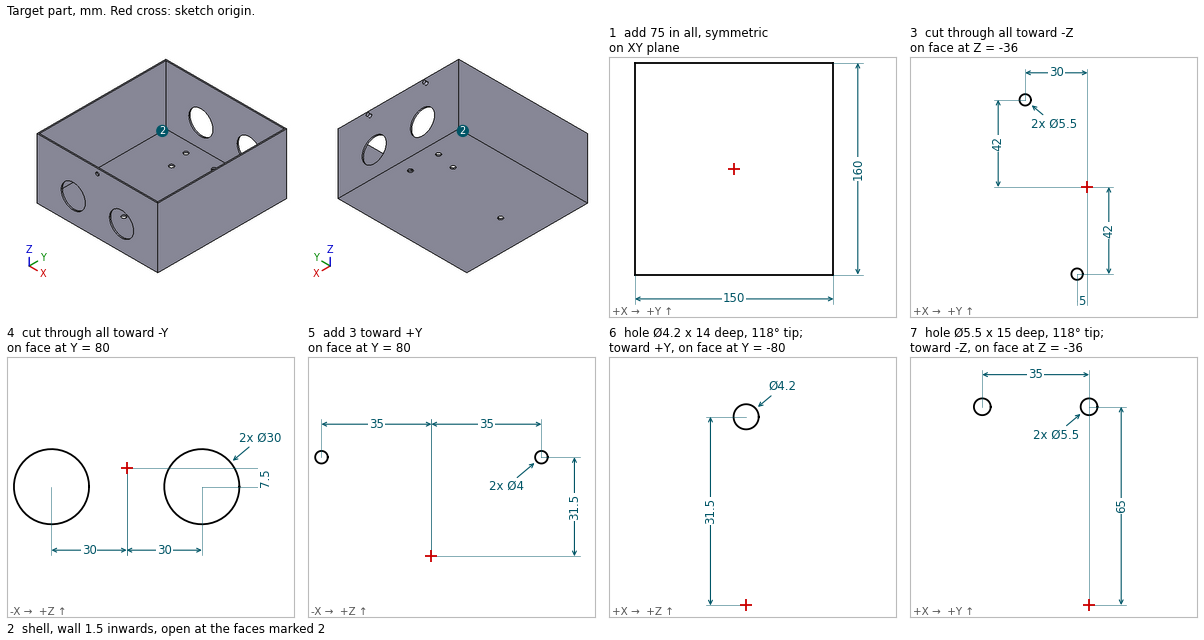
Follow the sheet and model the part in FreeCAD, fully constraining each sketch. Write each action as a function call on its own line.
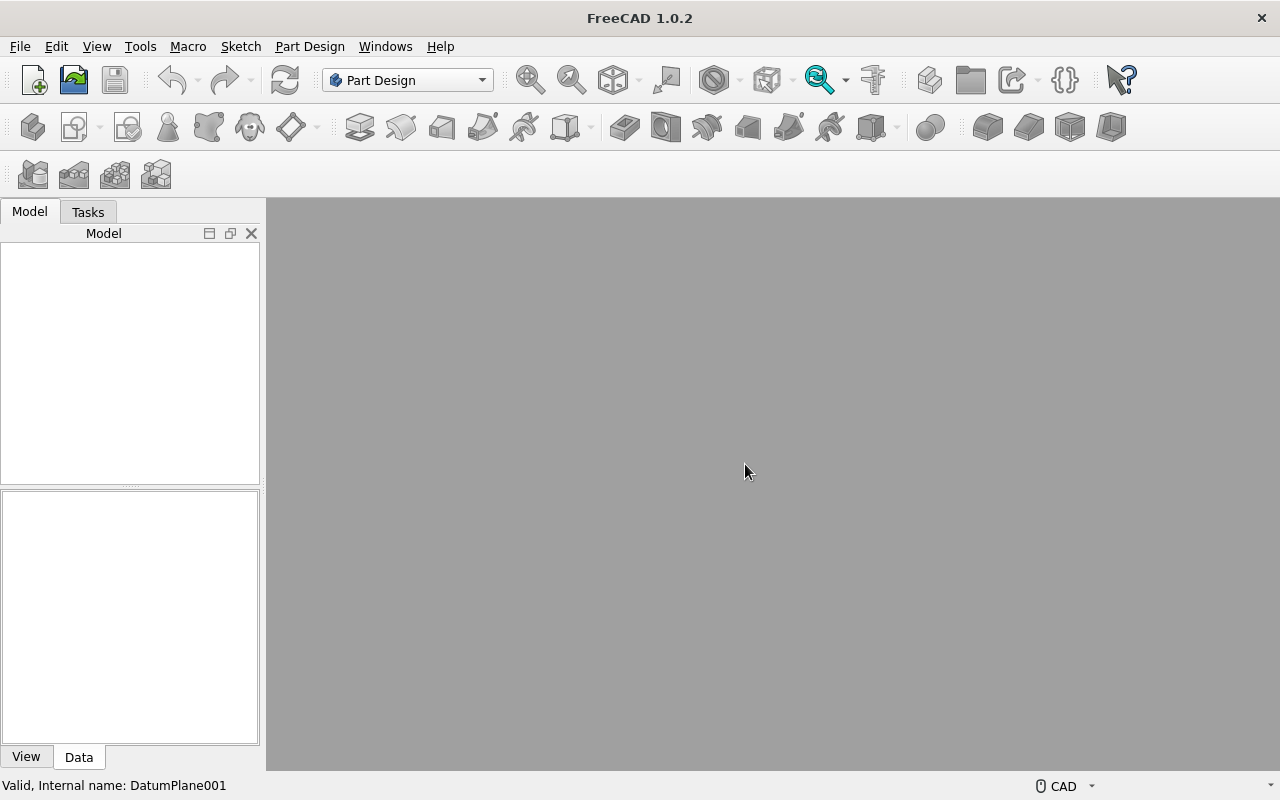
key(ctrl+n)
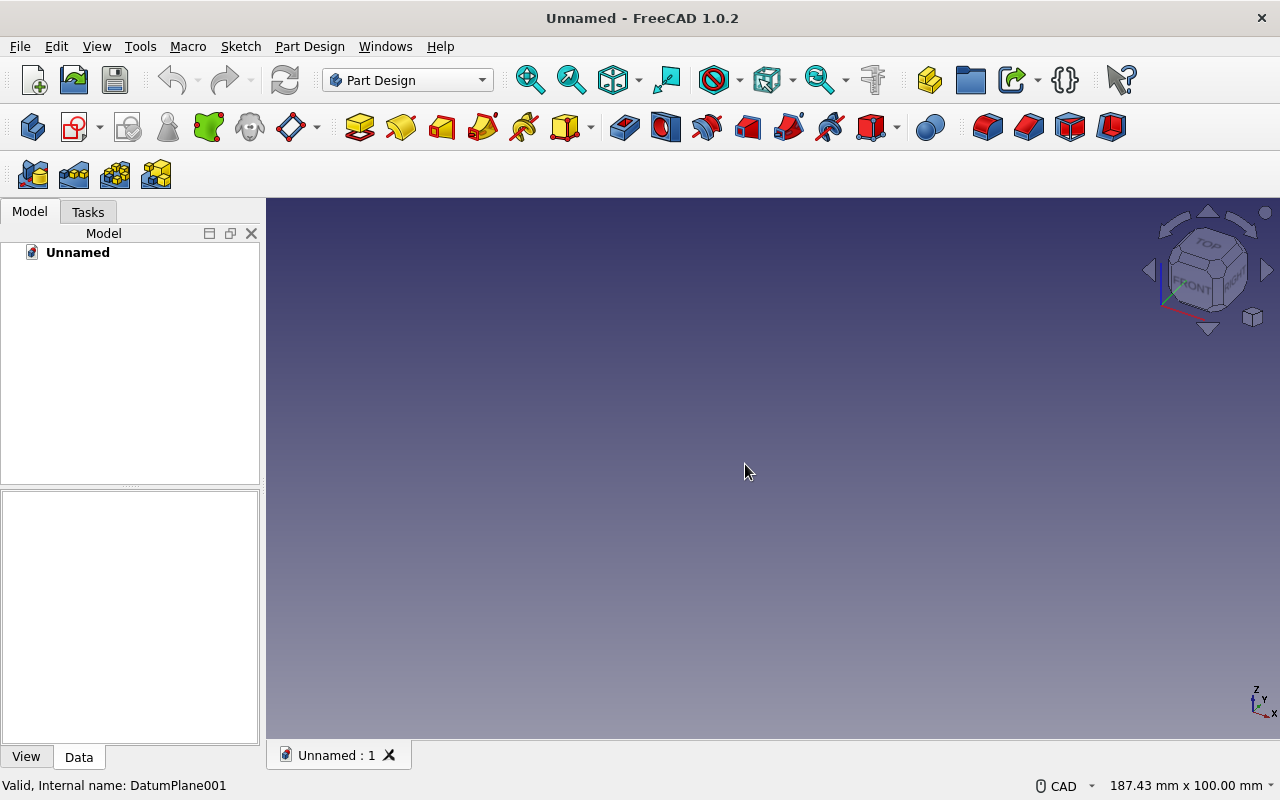
click(74, 128)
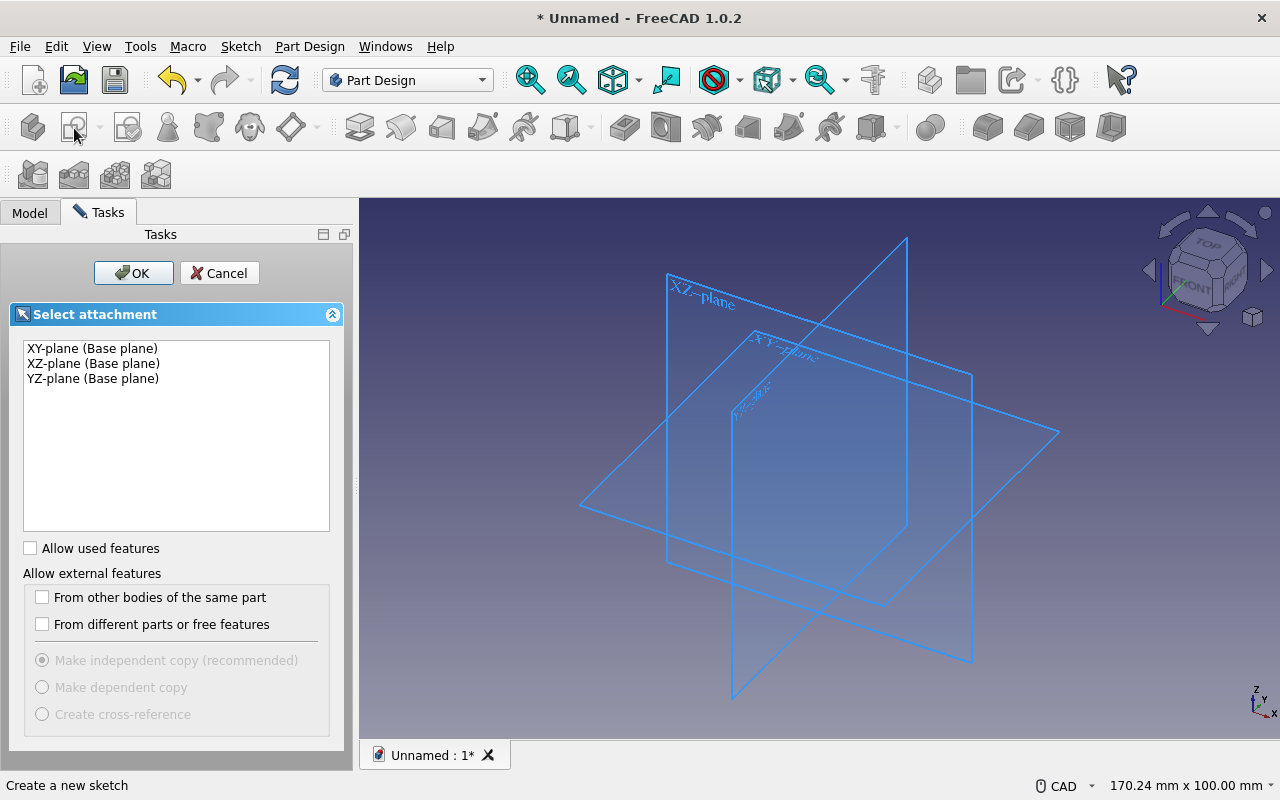
click(84, 348)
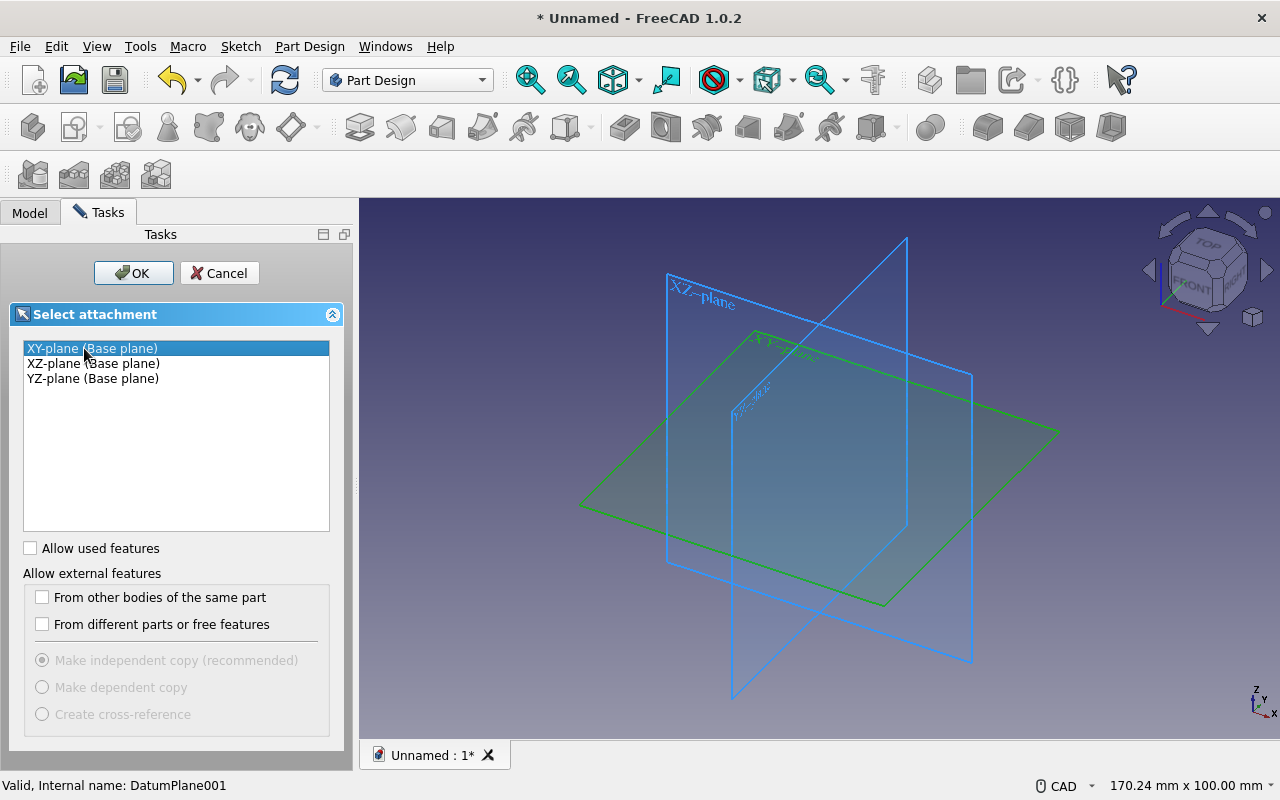
click(134, 273)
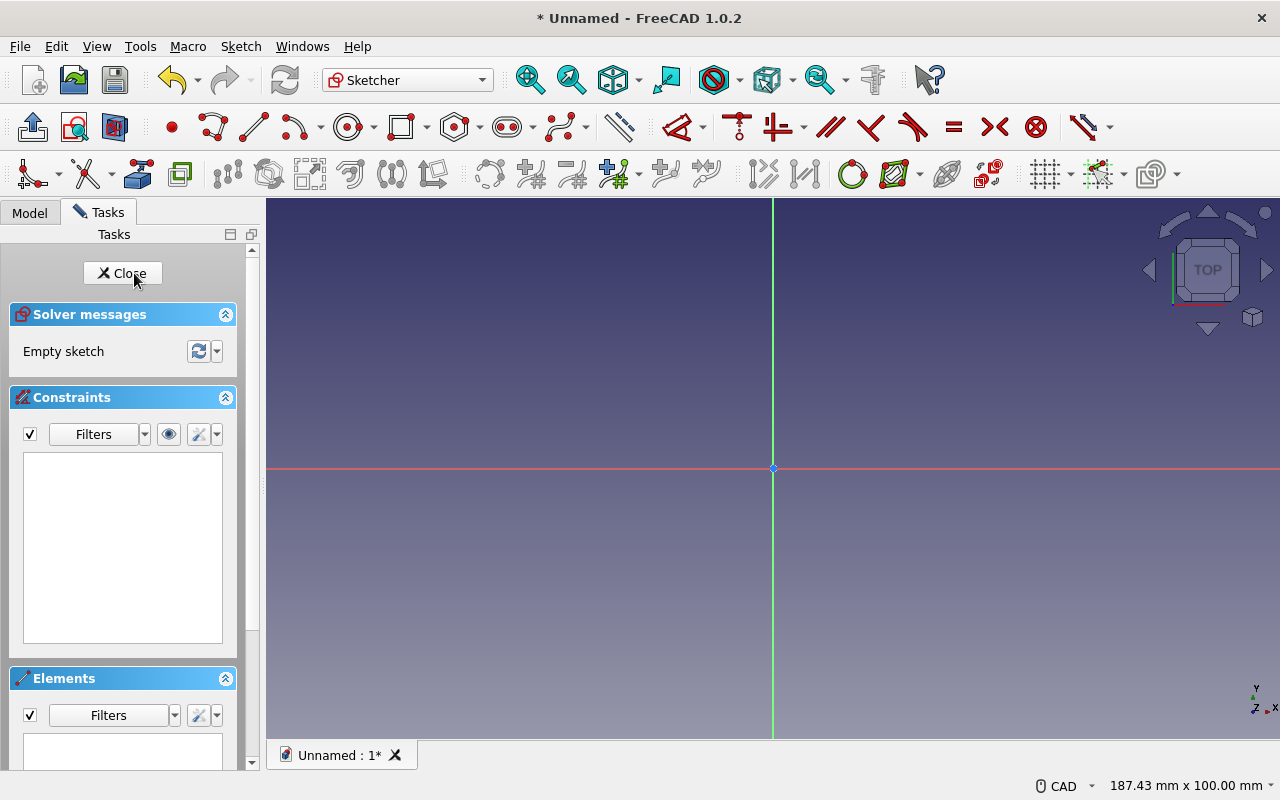
scroll(665, 469, down, 5)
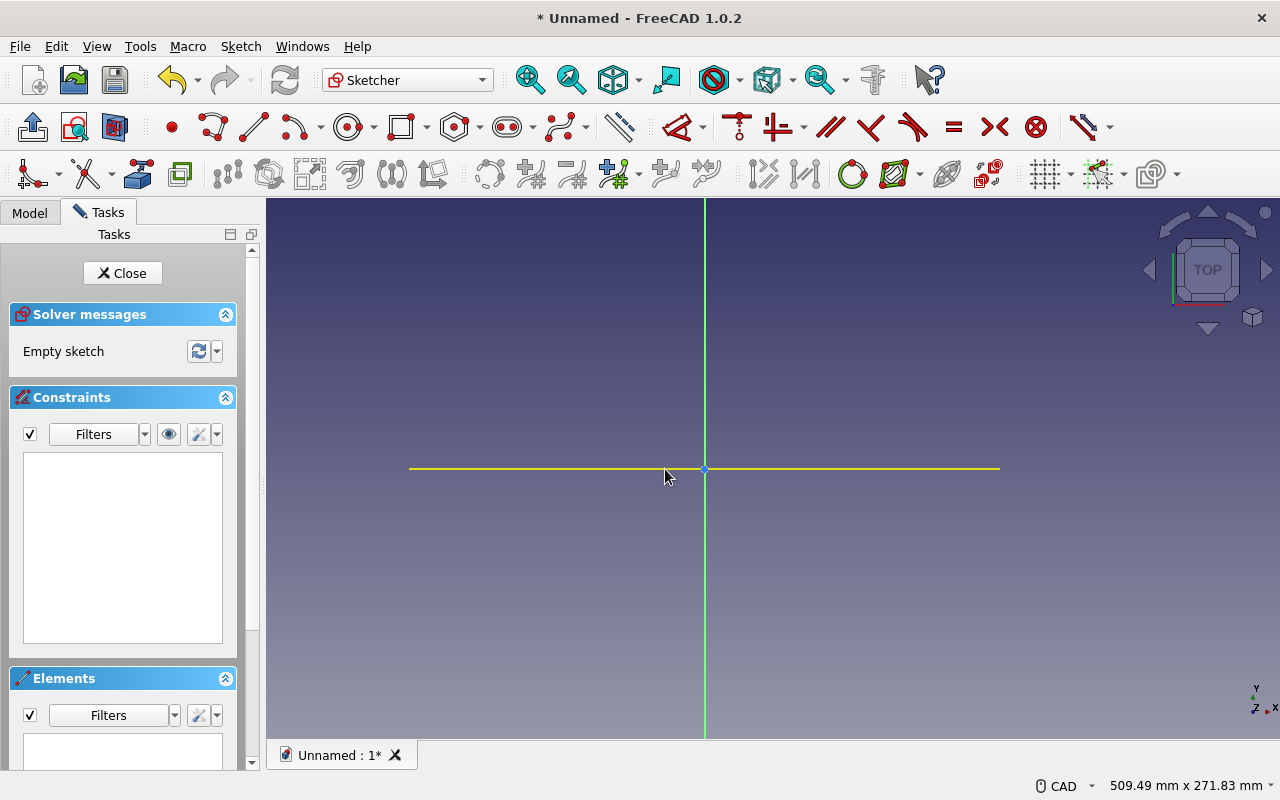
key(g)
key(v)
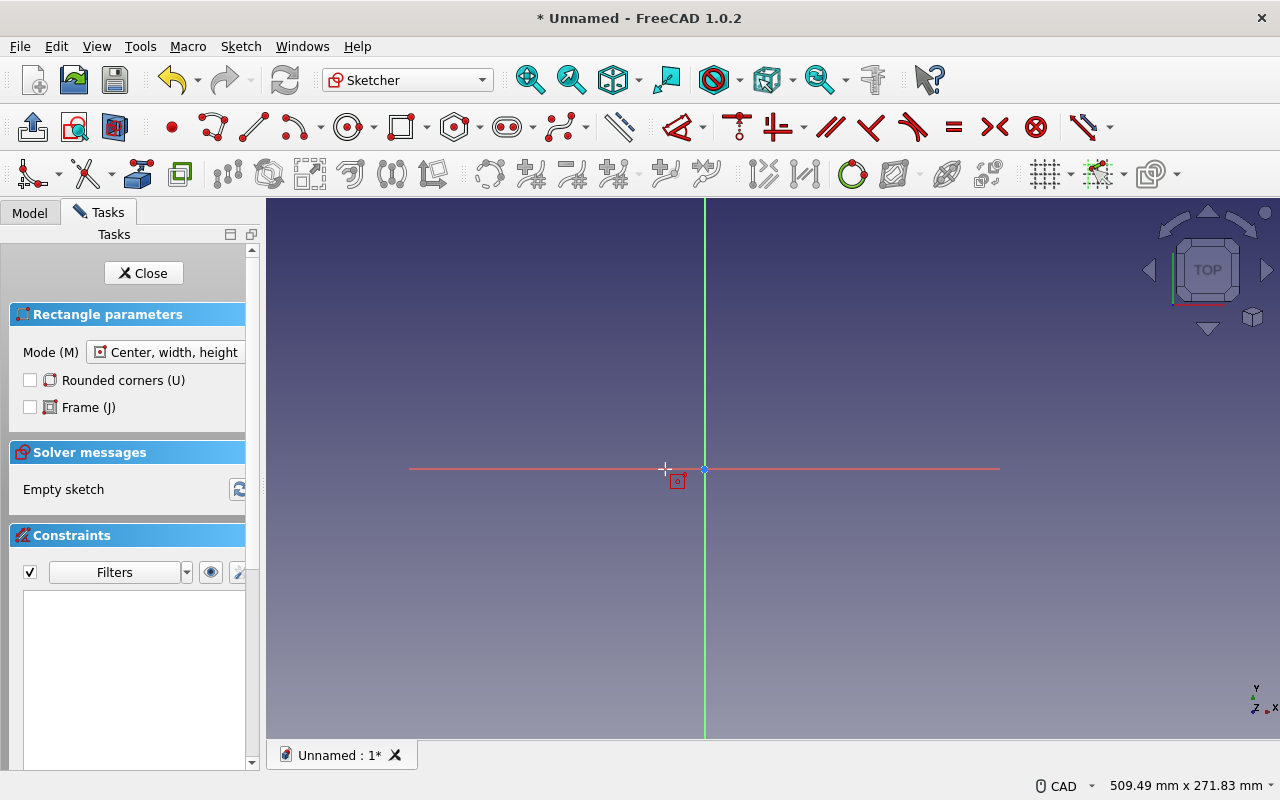
click(705, 469)
move(854, 310)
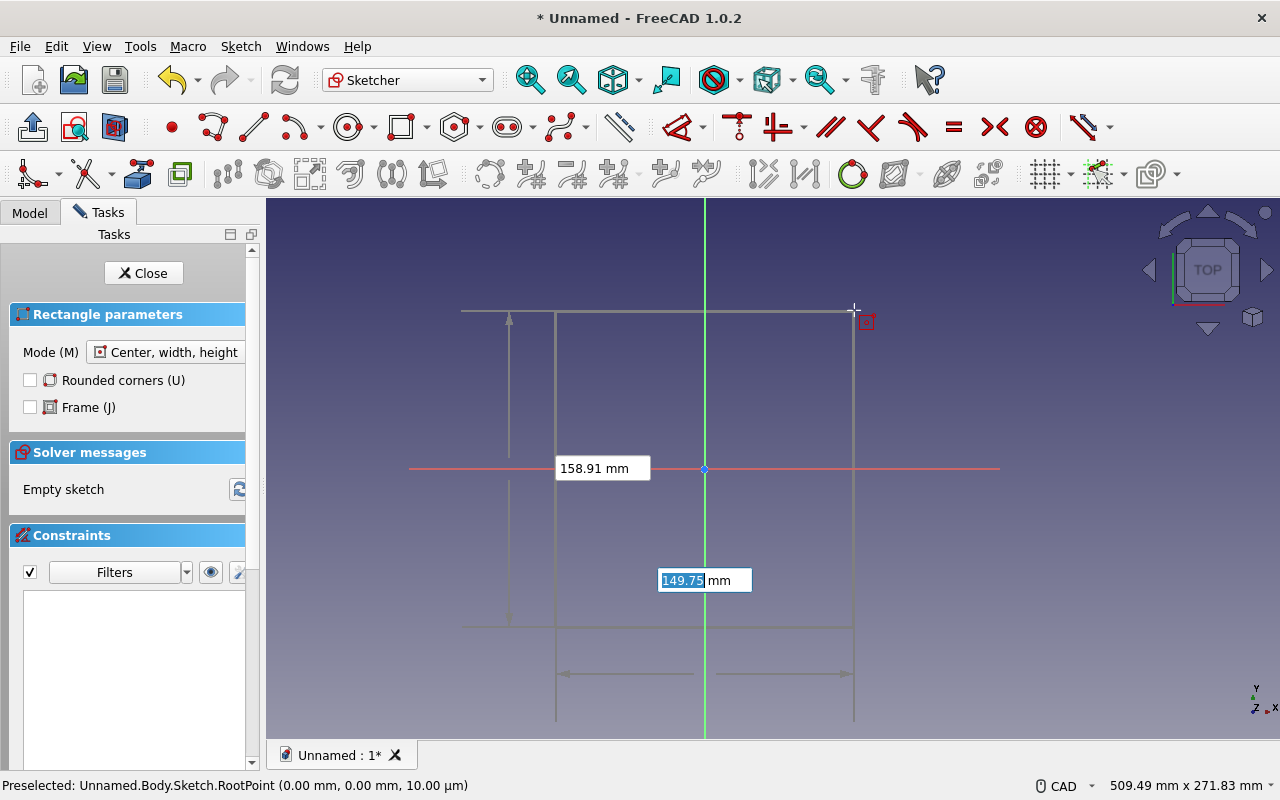
text(150)
key(Tab)
text(160)
key(Return)
key(Escape)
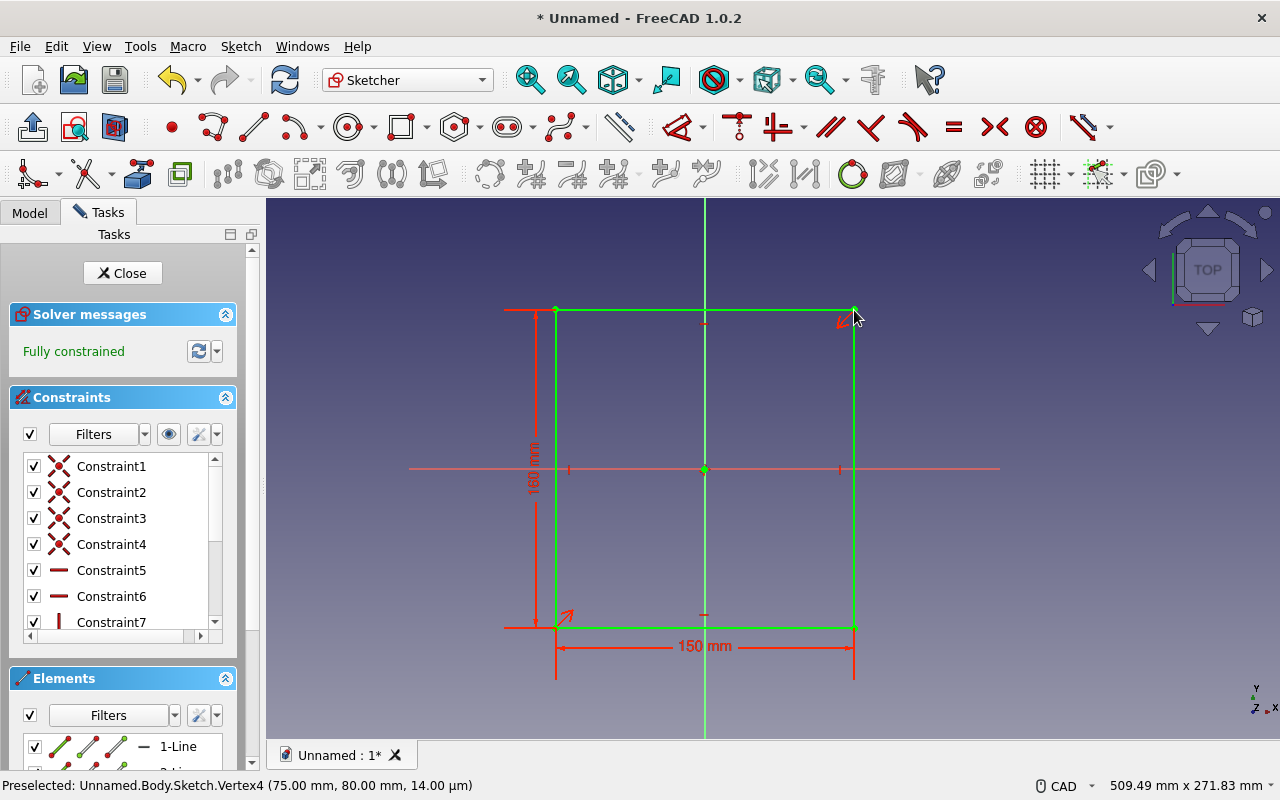
click(123, 273)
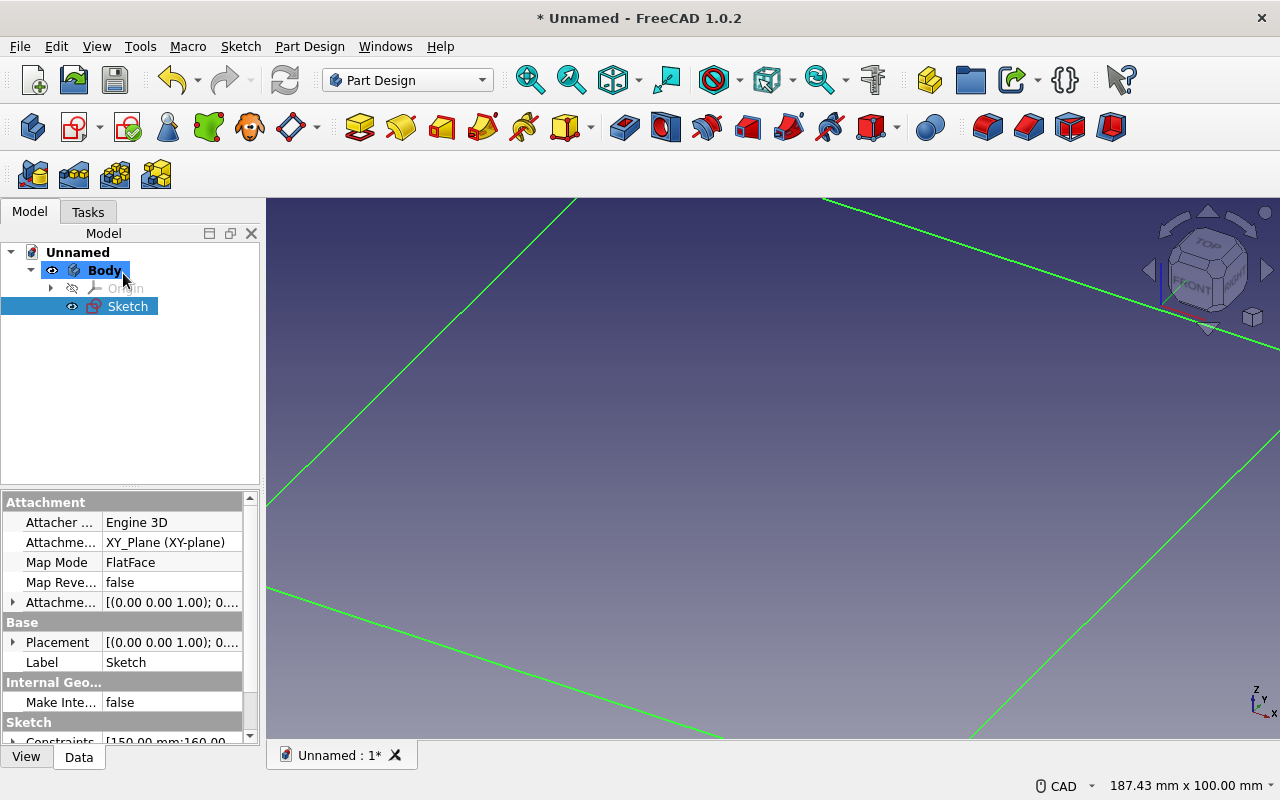
click(360, 128)